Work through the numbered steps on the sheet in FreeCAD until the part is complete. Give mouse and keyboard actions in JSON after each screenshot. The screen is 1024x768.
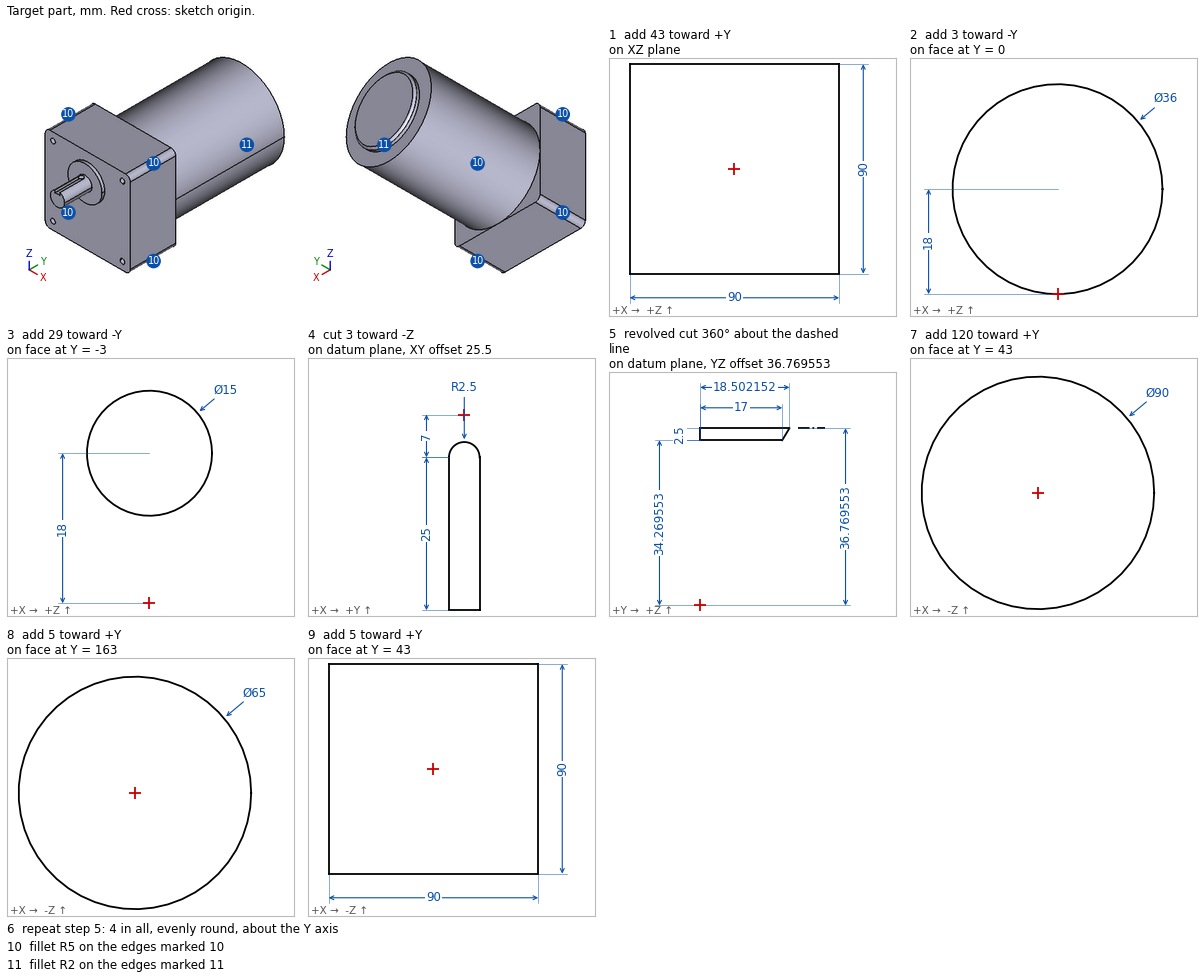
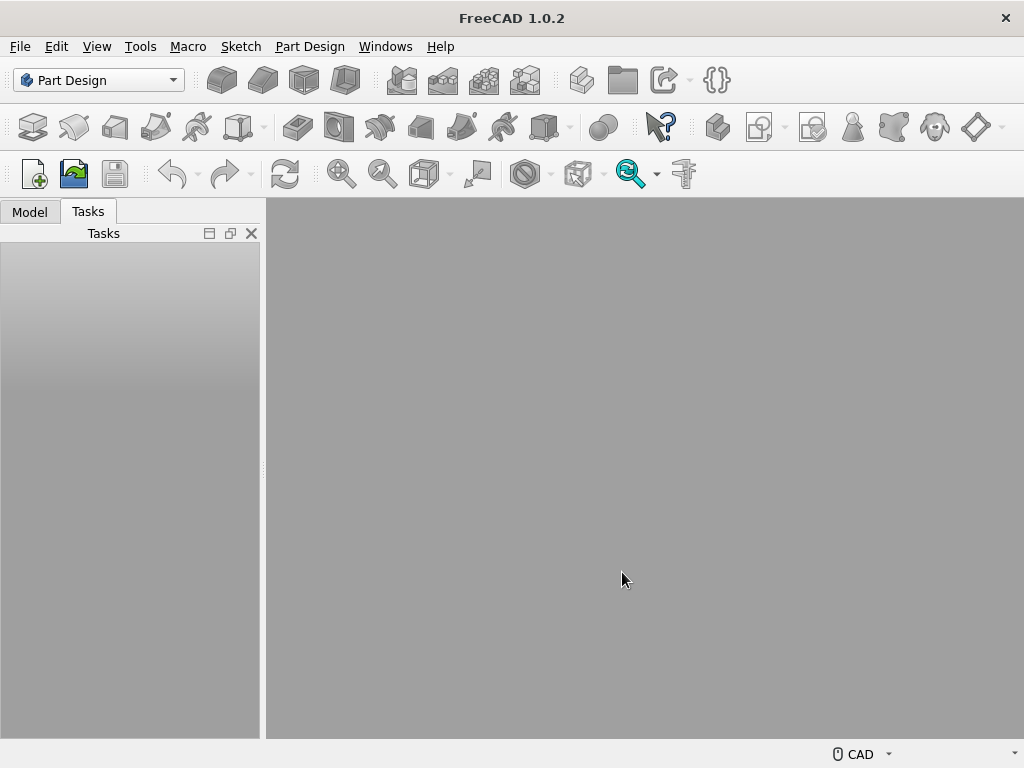
{"action": "left_click", "coordinate": [33, 174]}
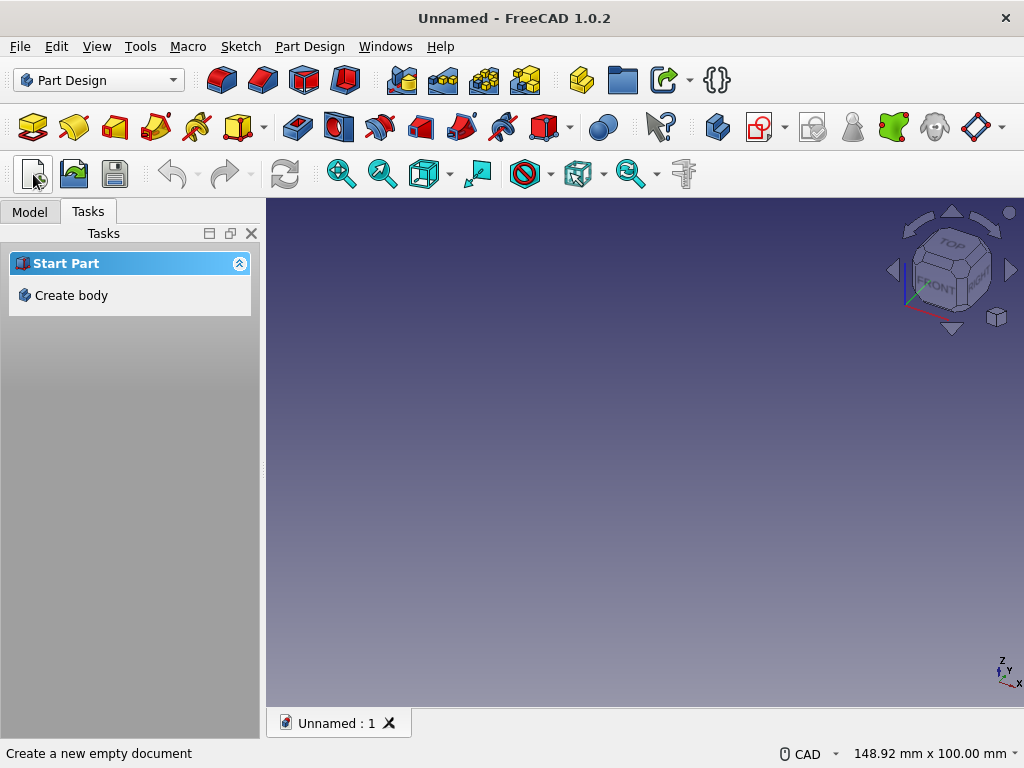
{"action": "left_click", "coordinate": [758, 128]}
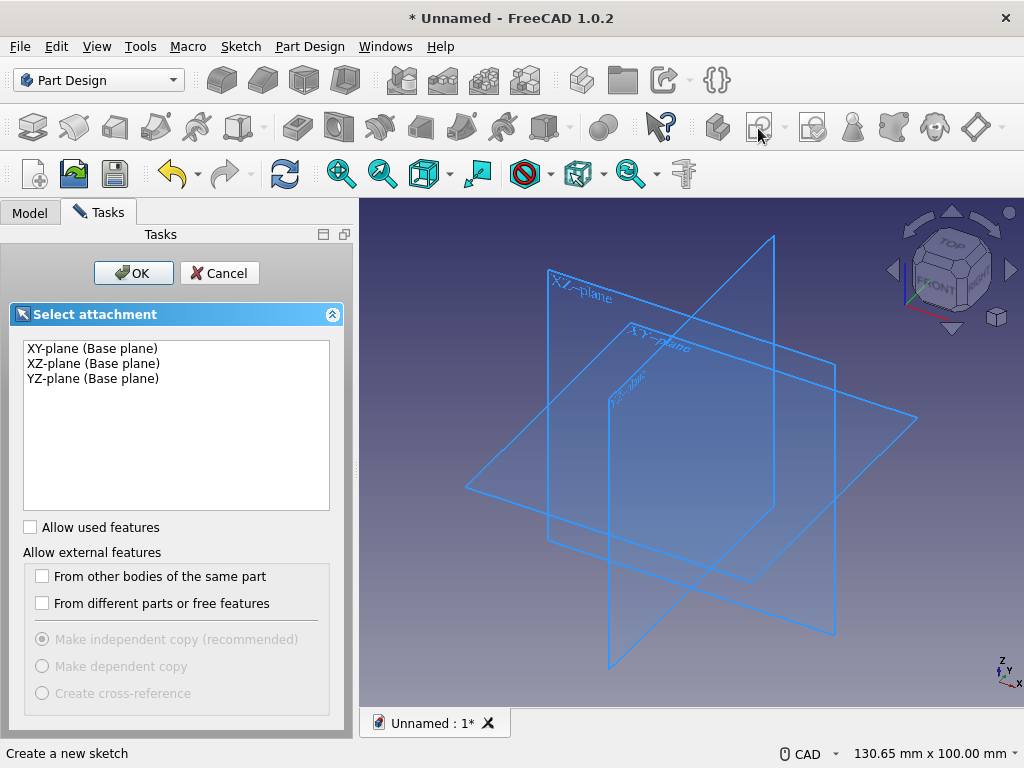
{"action": "left_click", "coordinate": [84, 364]}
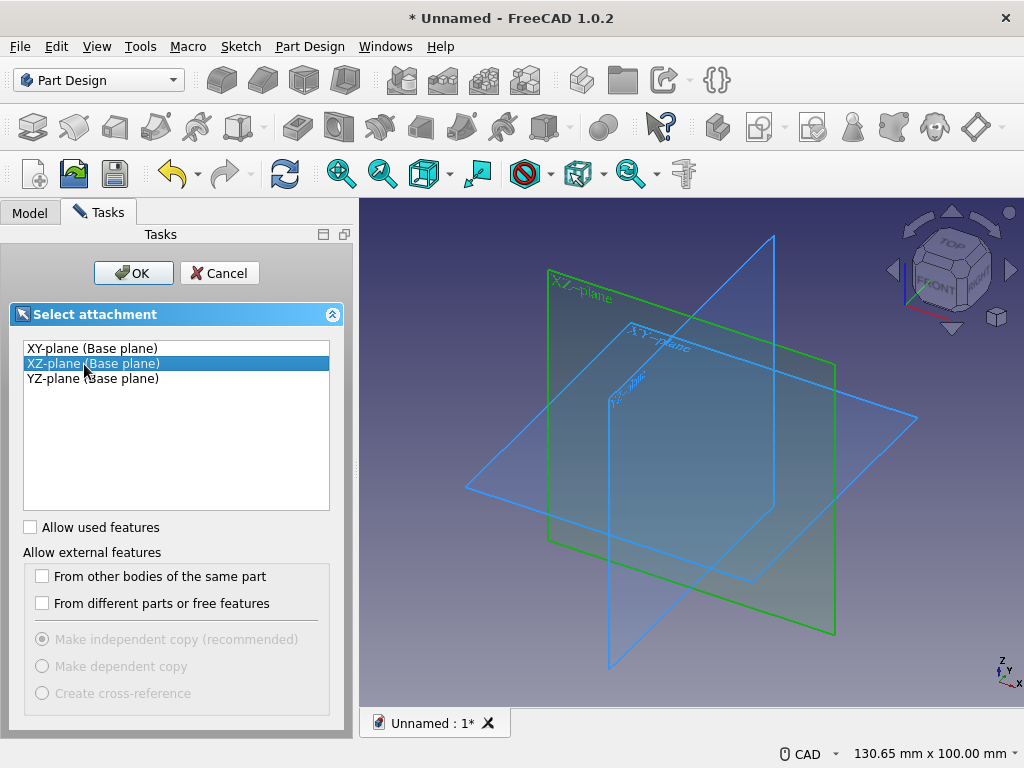
{"action": "left_click", "coordinate": [134, 273]}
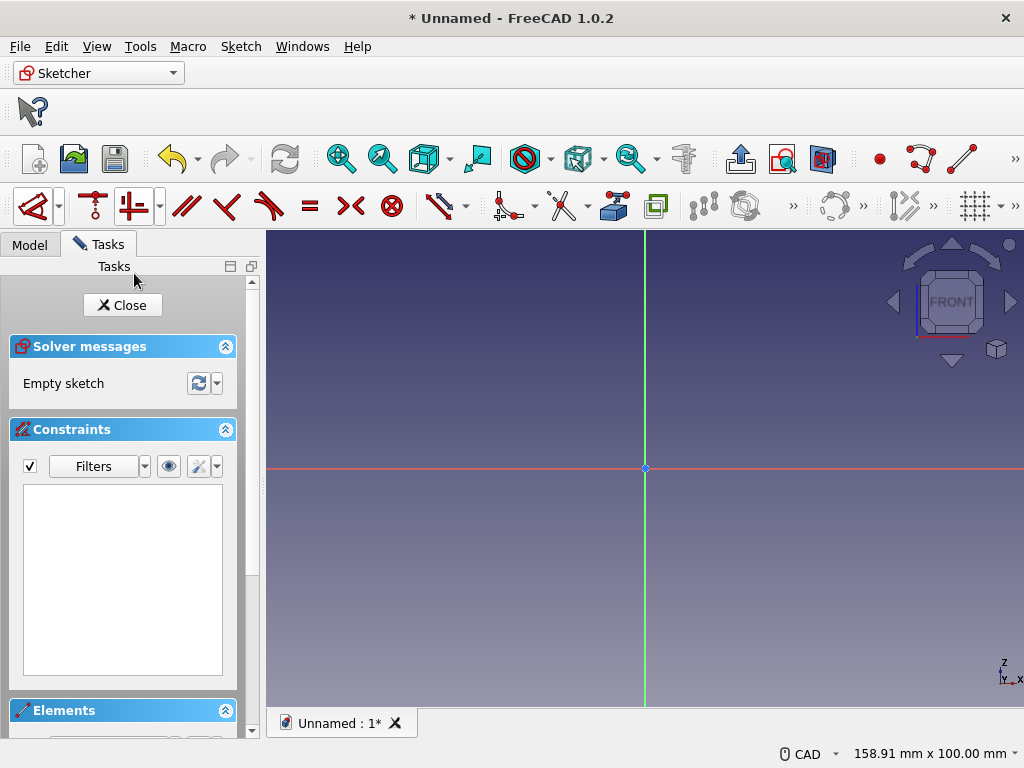
{"action": "scroll", "coordinate": [437, 468], "scroll_direction": "down", "scroll_amount": 2}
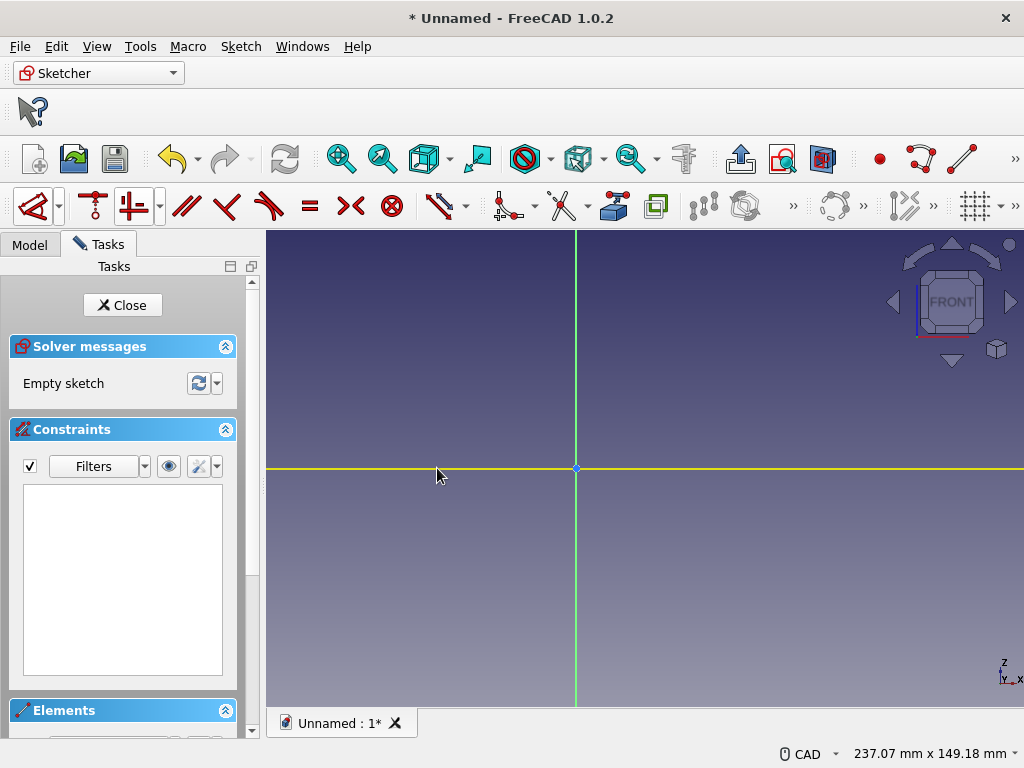
{"action": "key", "text": "g v"}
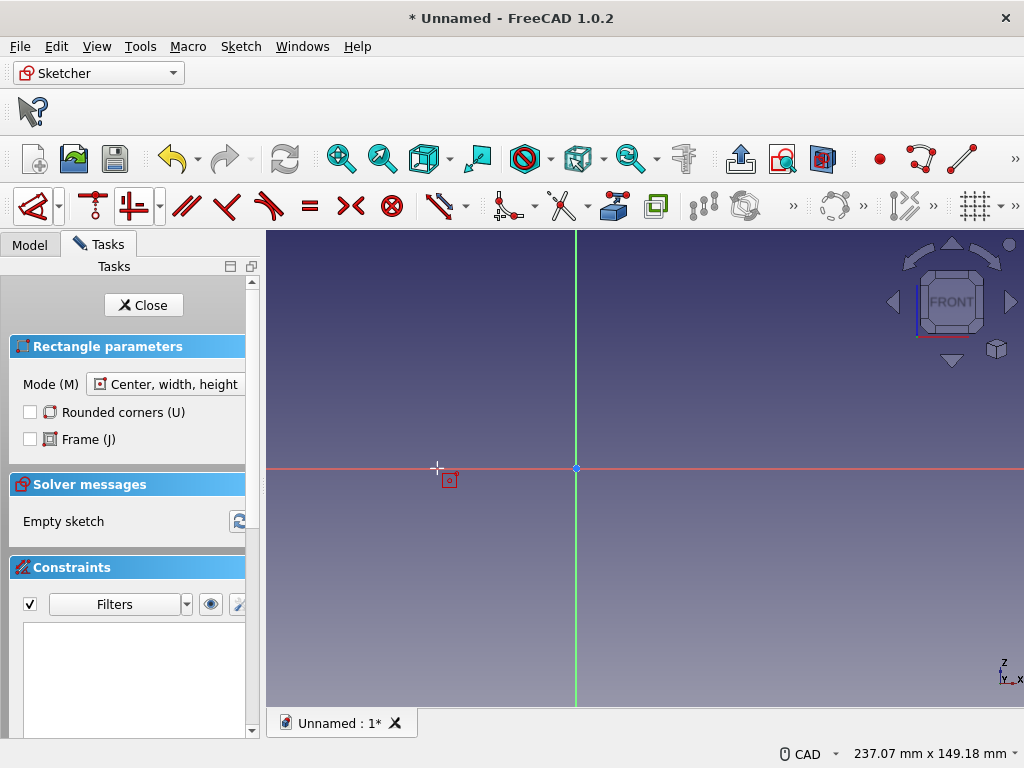
{"action": "left_click", "coordinate": [577, 468]}
{"action": "mouse_move", "coordinate": [720, 325]}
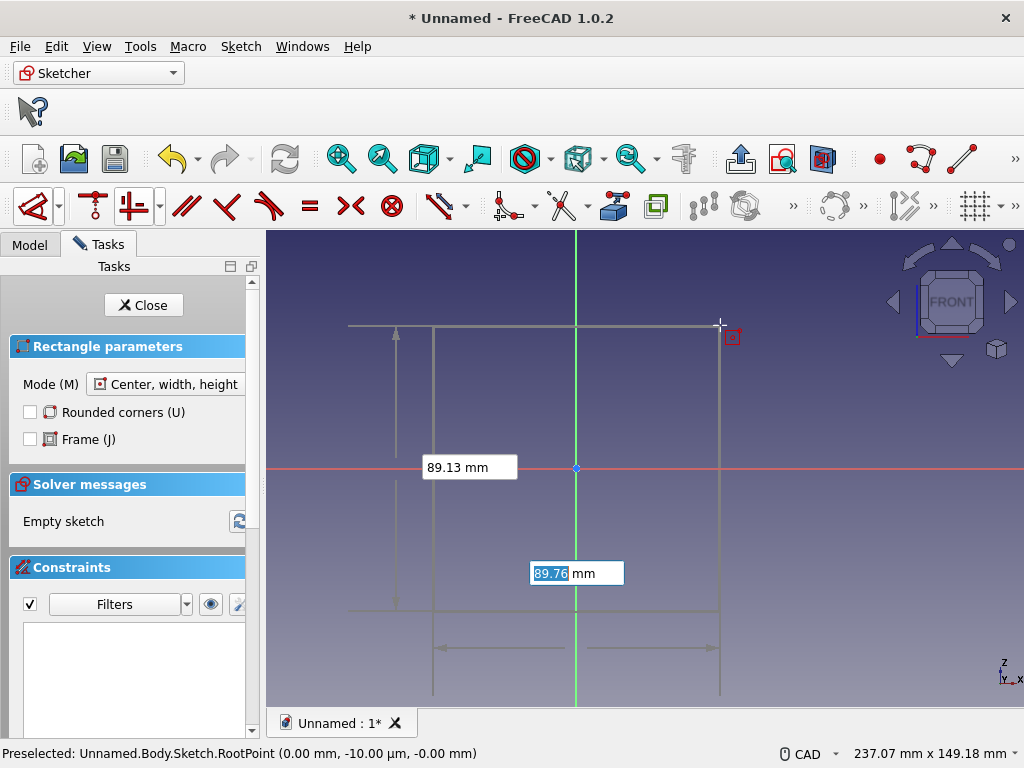
{"action": "type", "text": "90"}
{"action": "key", "text": "Tab"}
{"action": "type", "text": "90"}
{"action": "key", "text": "Return"}
{"action": "key", "text": "Escape"}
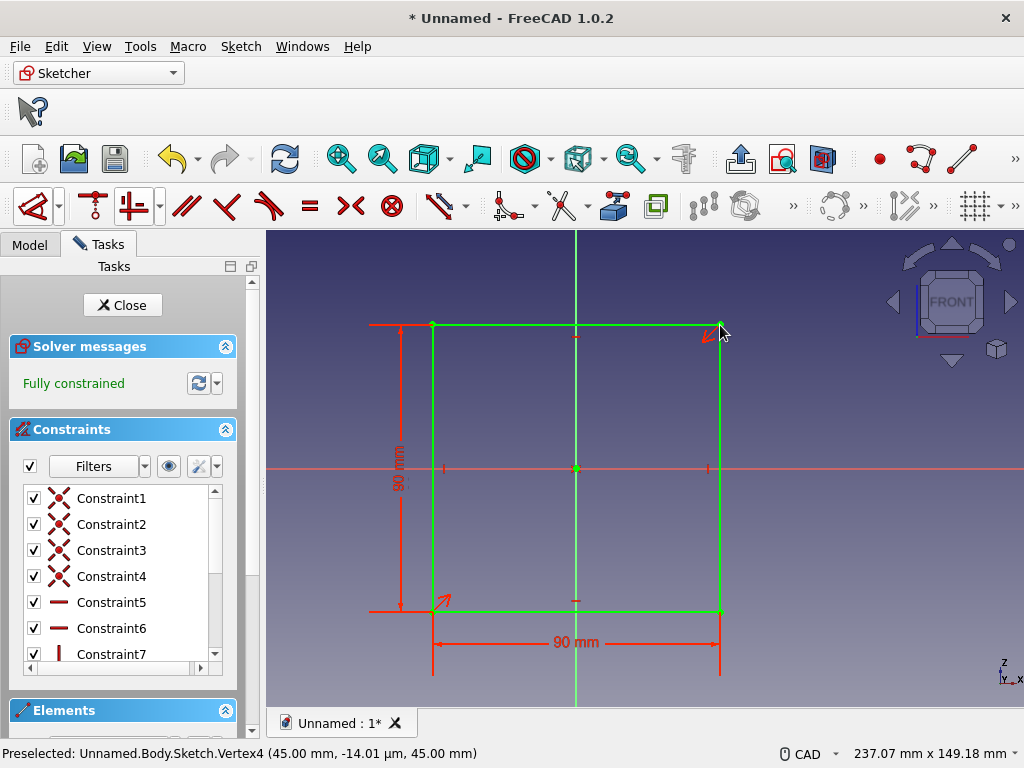
{"action": "left_click", "coordinate": [123, 305]}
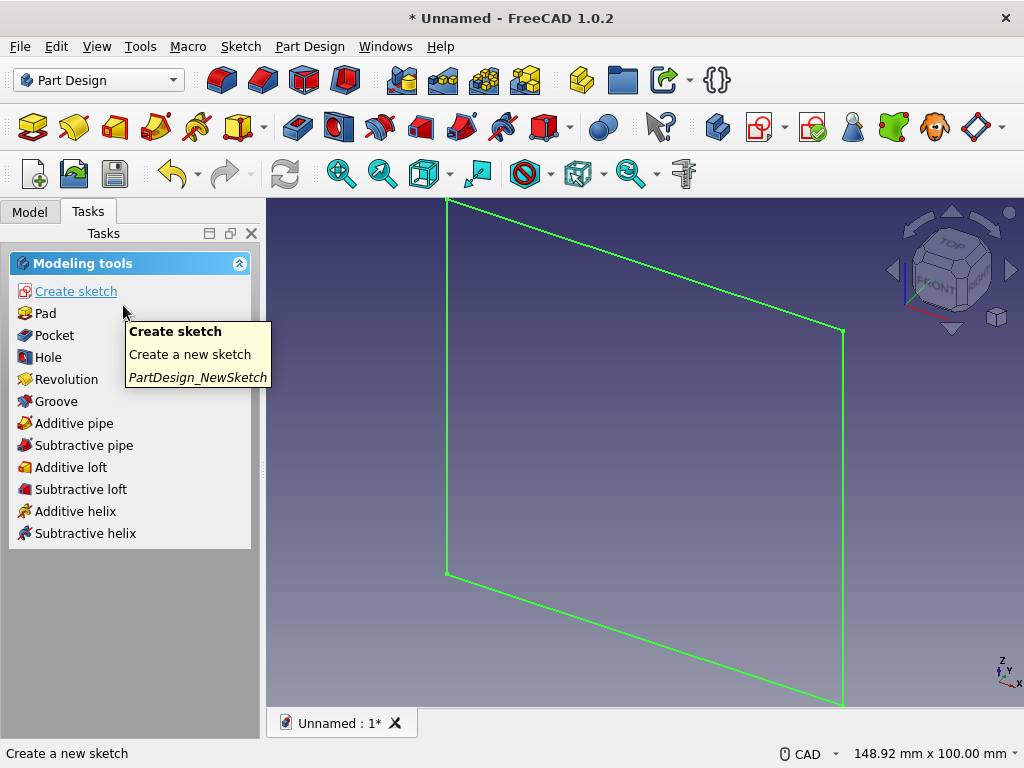
{"action": "left_click", "coordinate": [33, 128]}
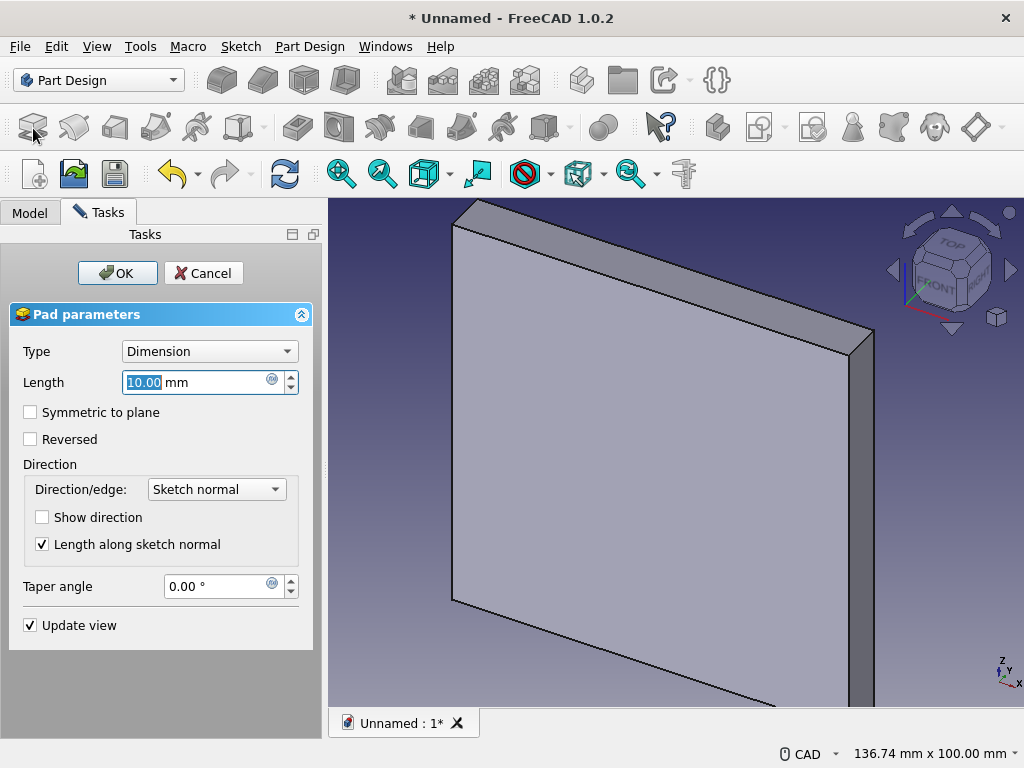
{"action": "type", "text": "43"}
{"action": "key", "text": "Tab"}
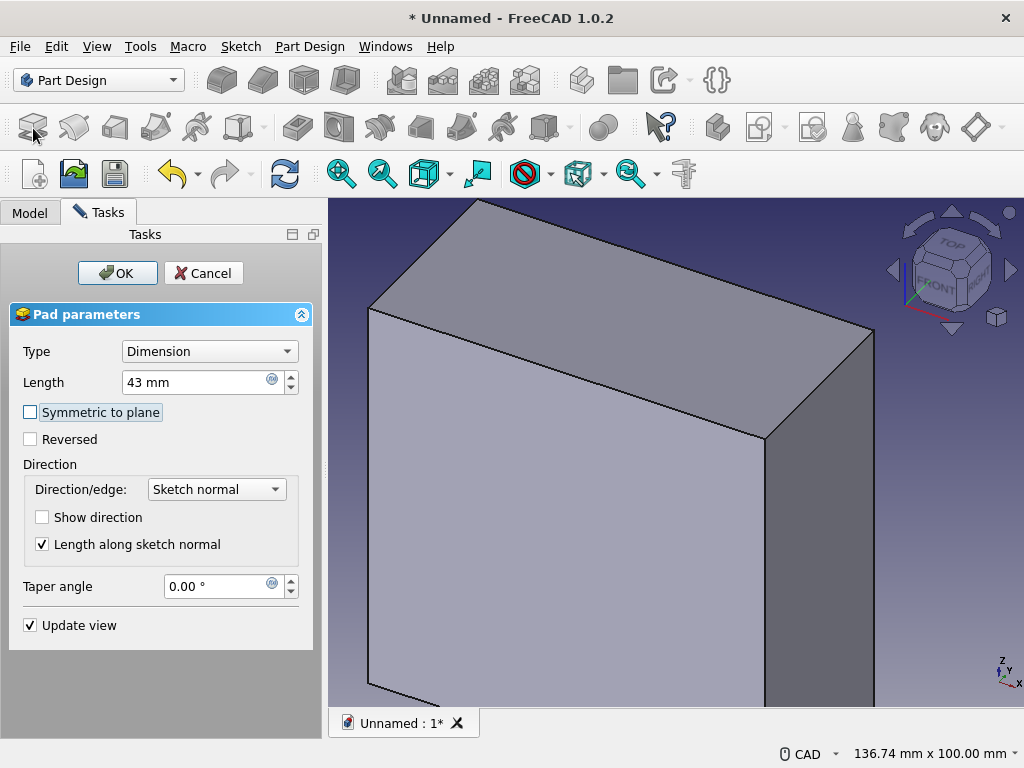
{"action": "left_click", "coordinate": [31, 439]}